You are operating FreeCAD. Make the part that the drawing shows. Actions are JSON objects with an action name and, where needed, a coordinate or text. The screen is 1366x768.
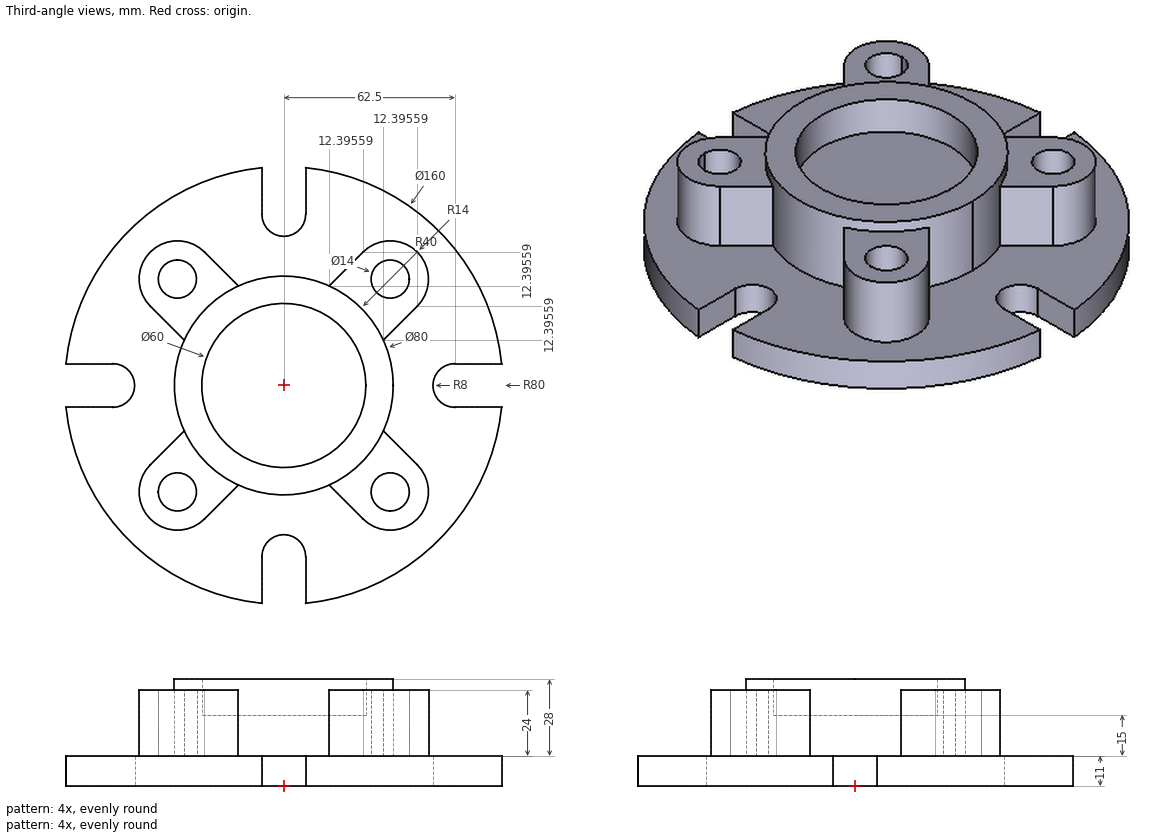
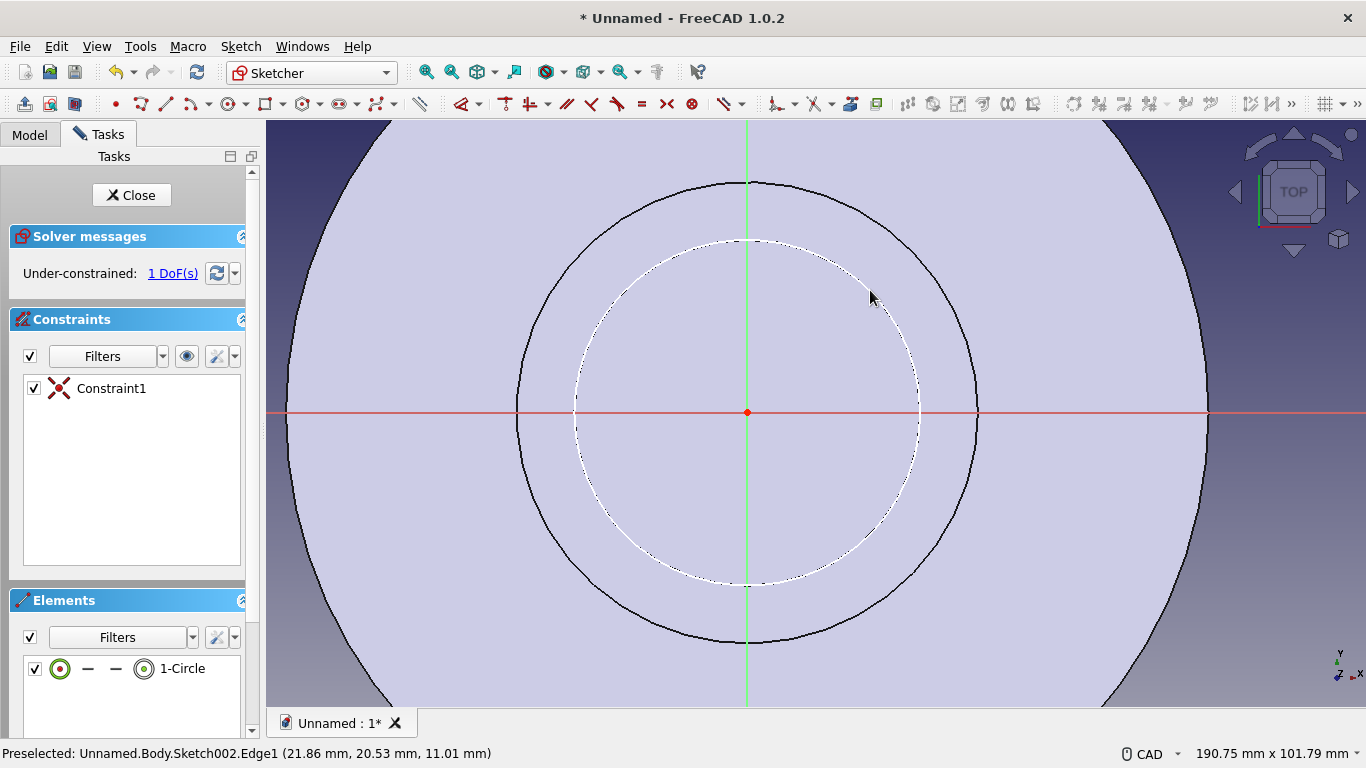
{"action": "key", "text": "d"}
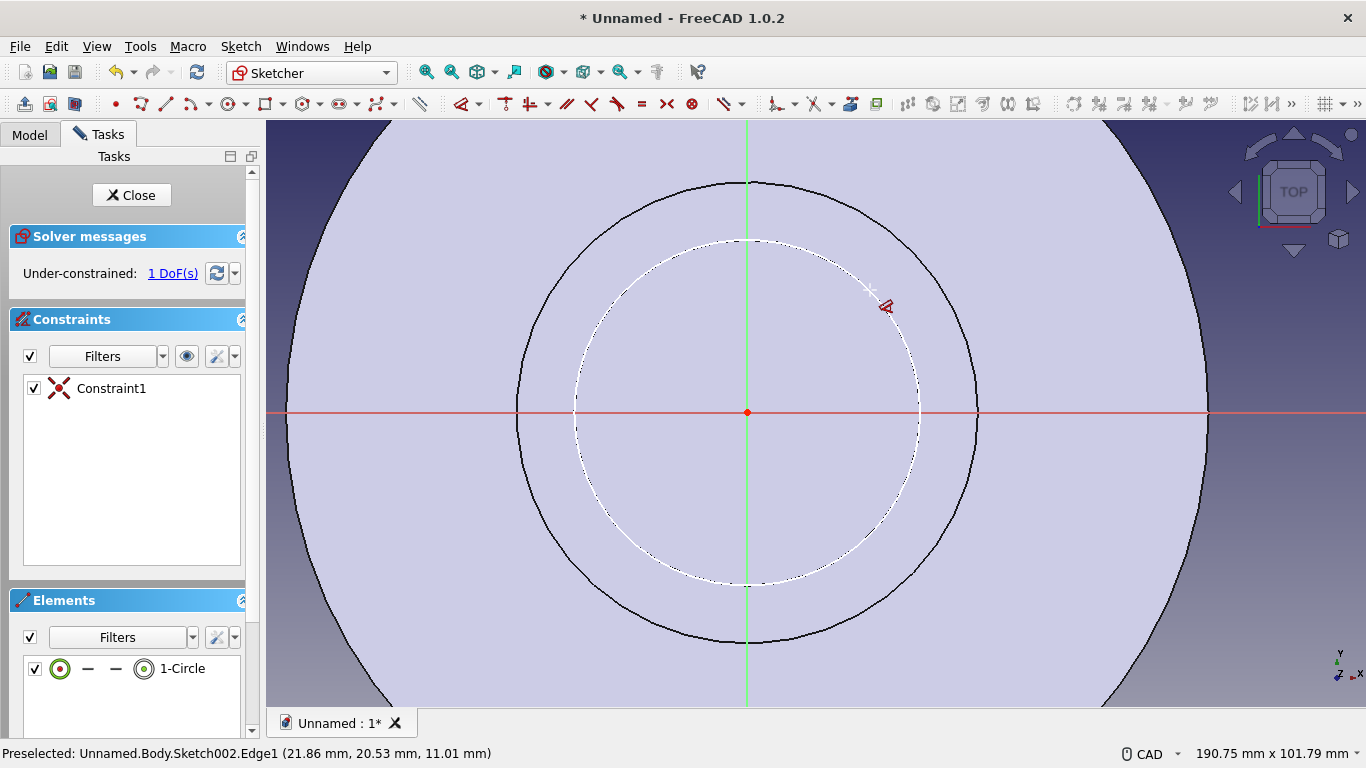
{"action": "left_click", "coordinate": [869, 290]}
{"action": "left_click", "coordinate": [892, 267]}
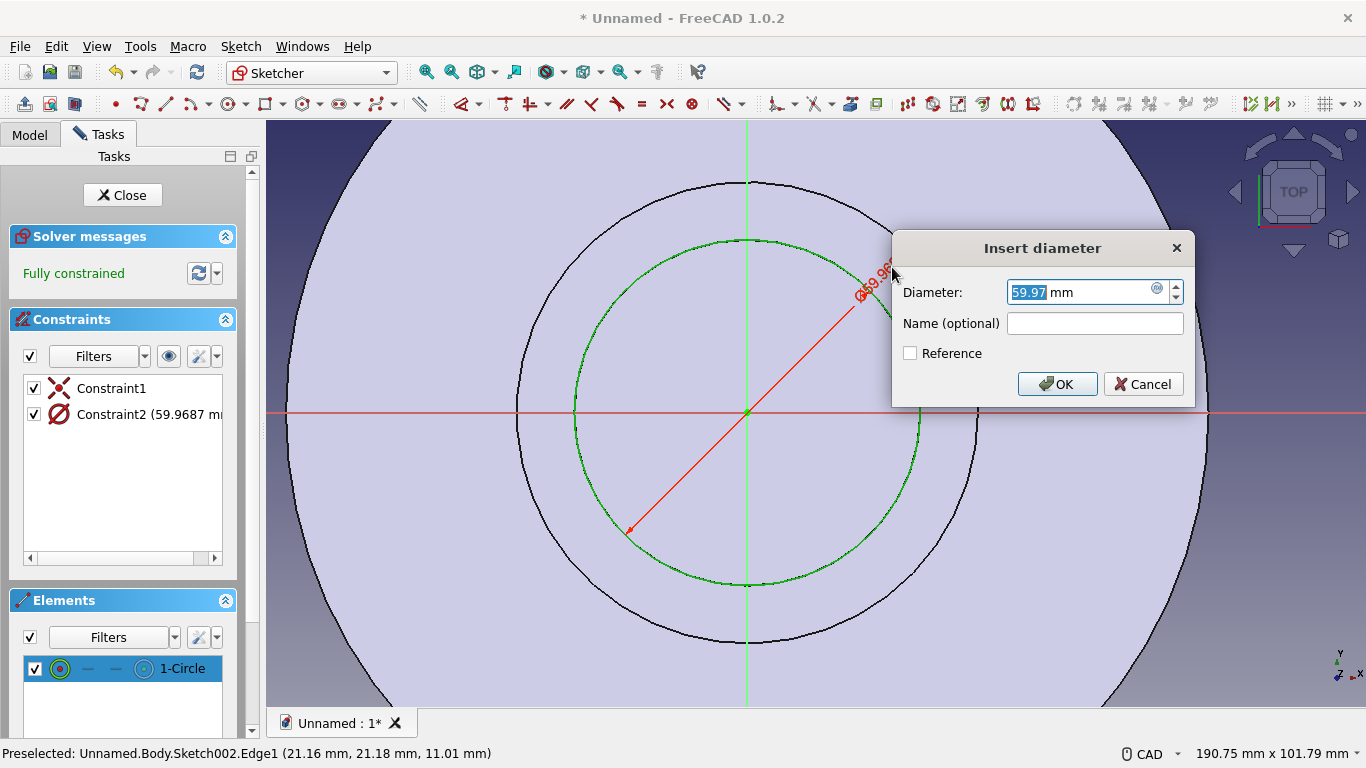
{"action": "type", "text": "60"}
{"action": "key", "text": "Return"}
{"action": "key", "text": "Escape"}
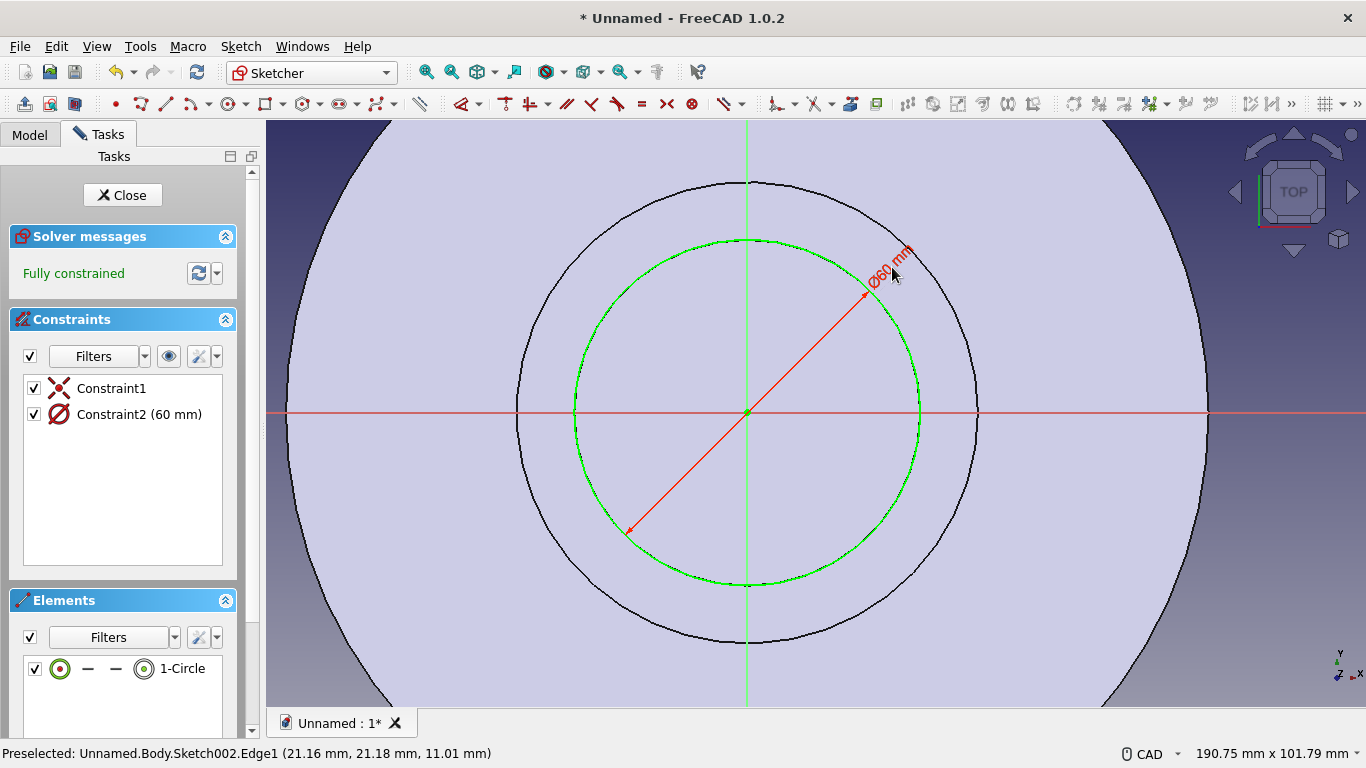
{"action": "left_click", "coordinate": [123, 195]}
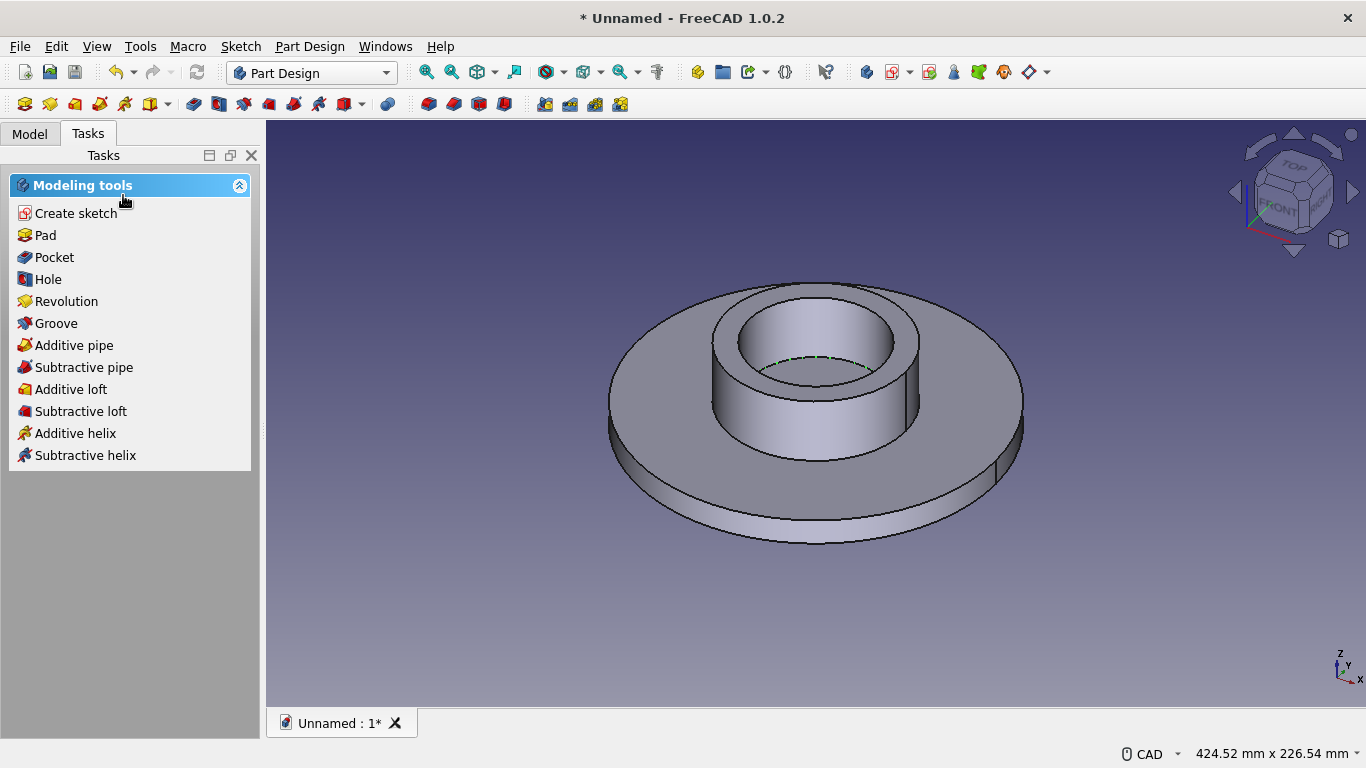
{"action": "left_click", "coordinate": [25, 104]}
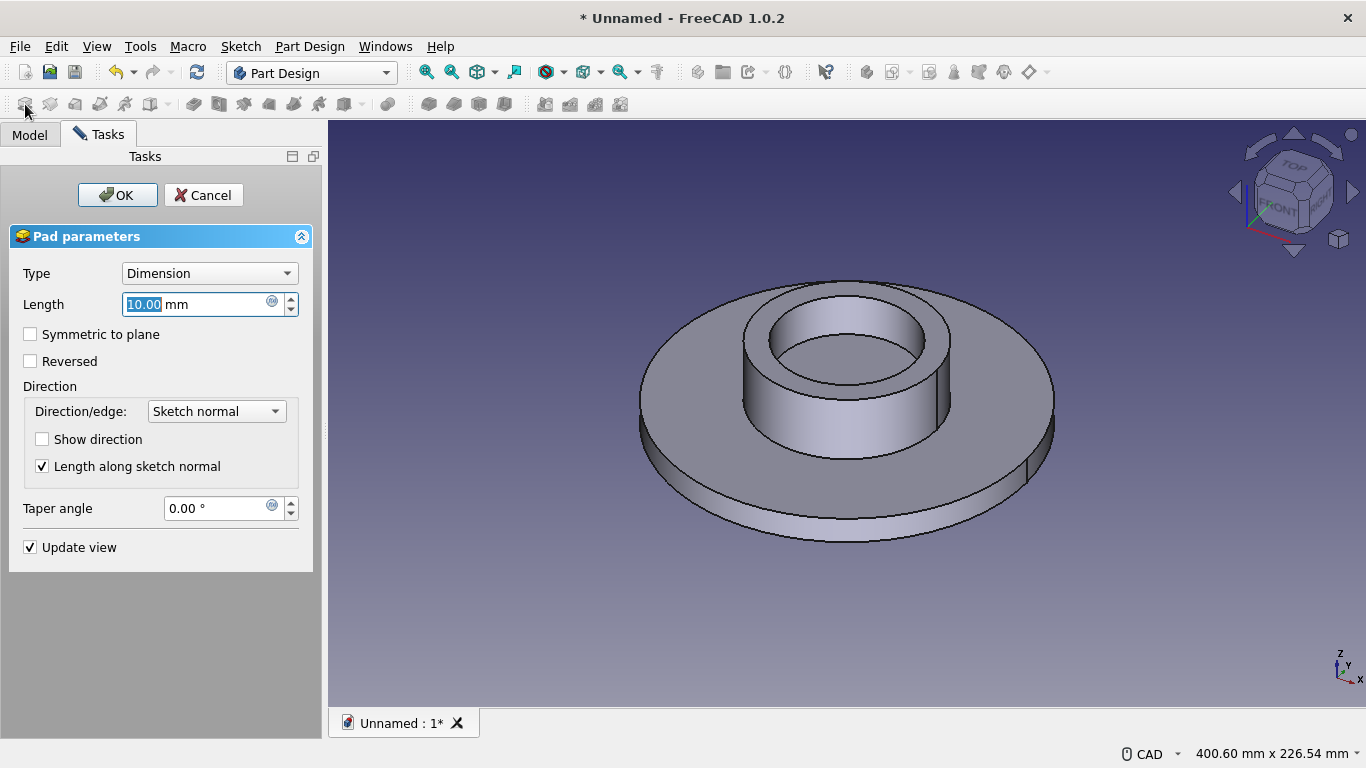
{"action": "type", "text": "15"}
{"action": "key", "text": "Tab"}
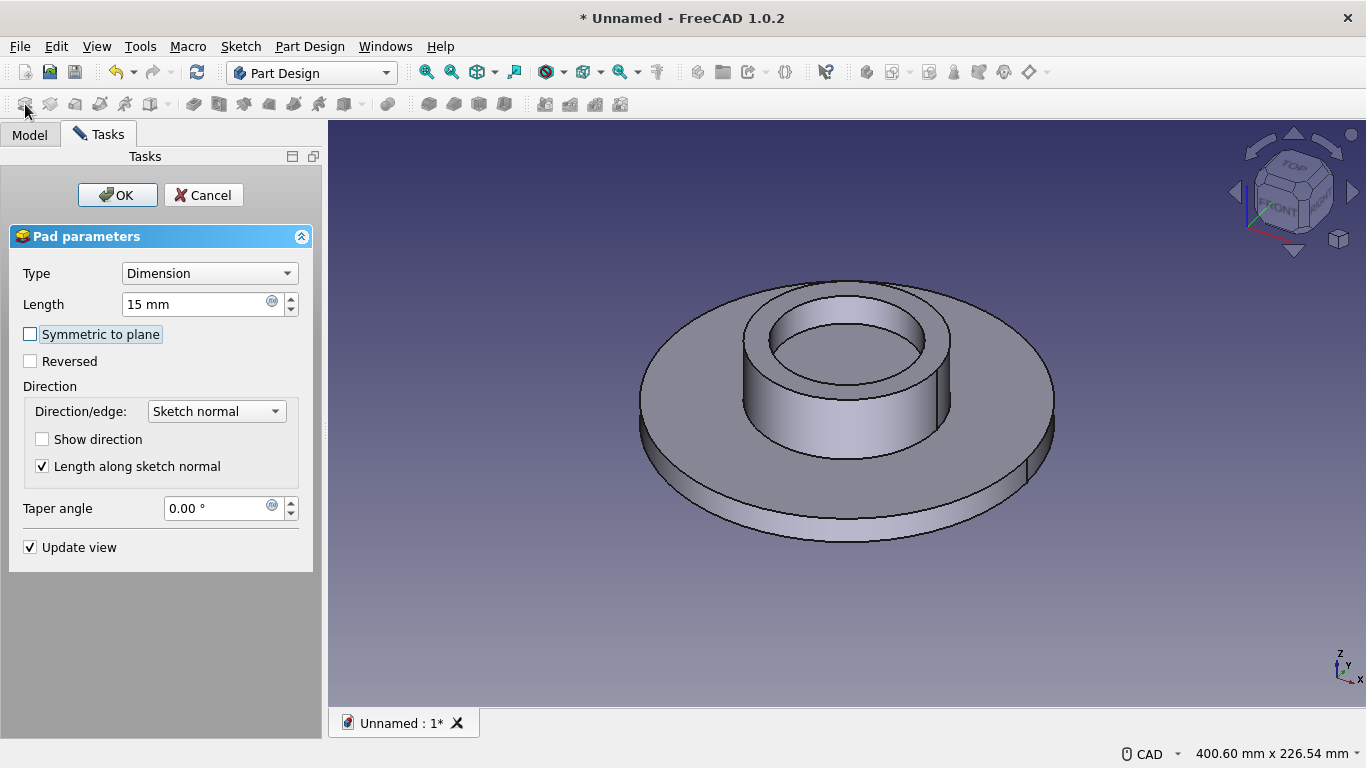
{"action": "left_click", "coordinate": [118, 195]}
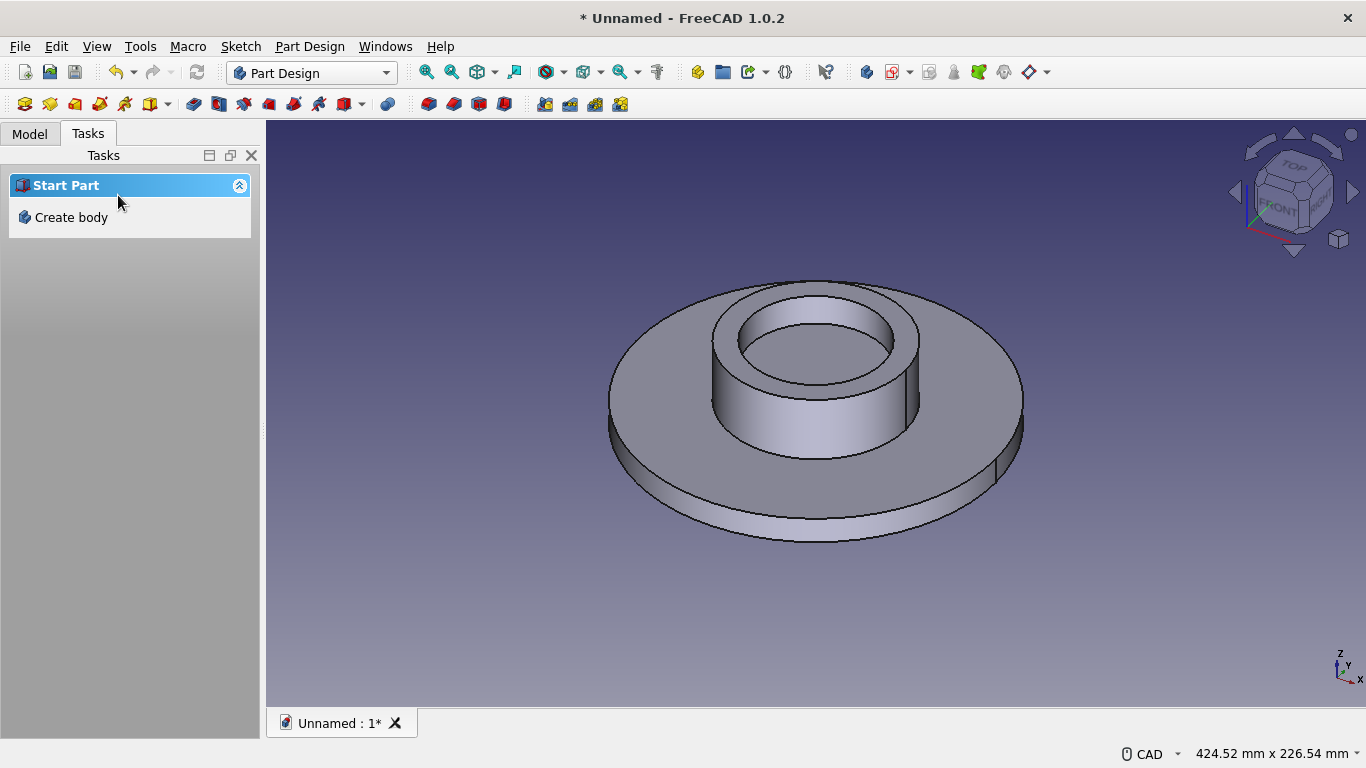
{"action": "left_click", "coordinate": [859, 492]}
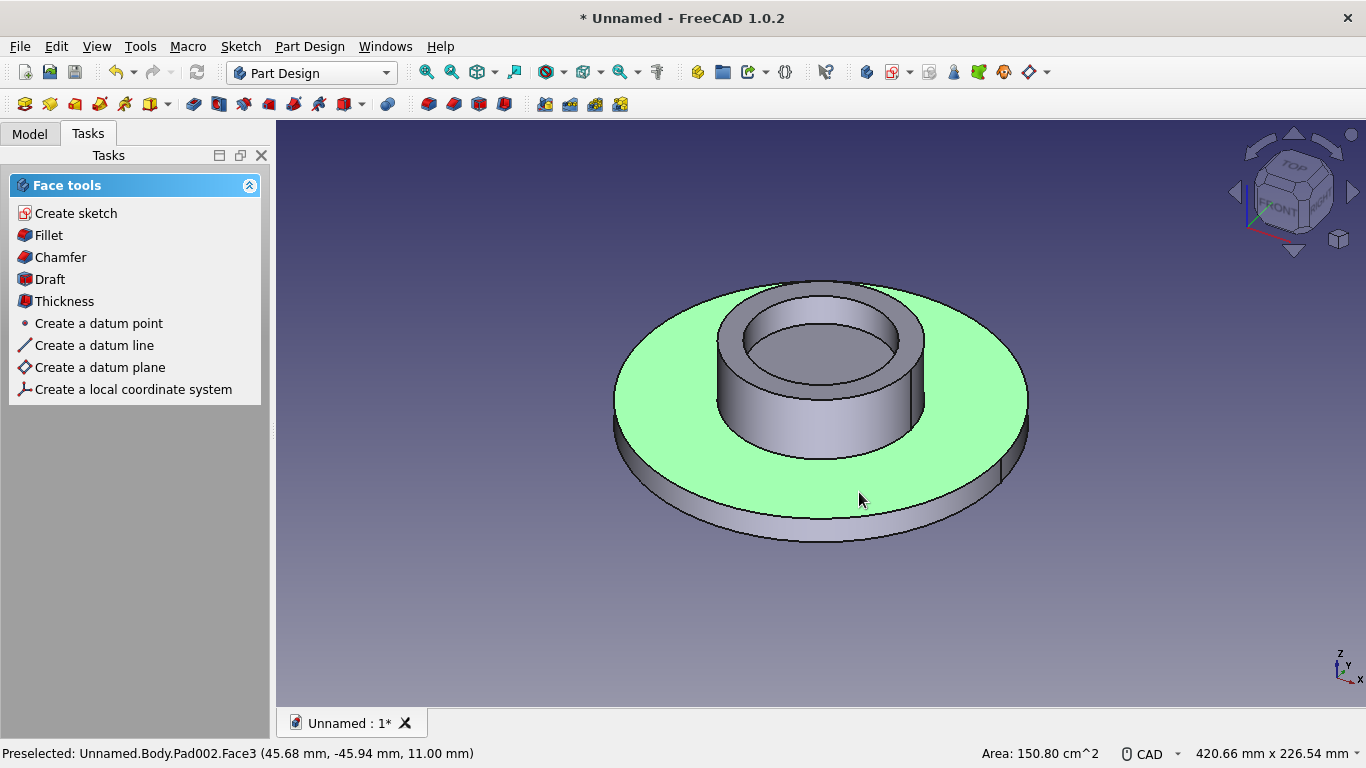
{"action": "left_click", "coordinate": [892, 72]}